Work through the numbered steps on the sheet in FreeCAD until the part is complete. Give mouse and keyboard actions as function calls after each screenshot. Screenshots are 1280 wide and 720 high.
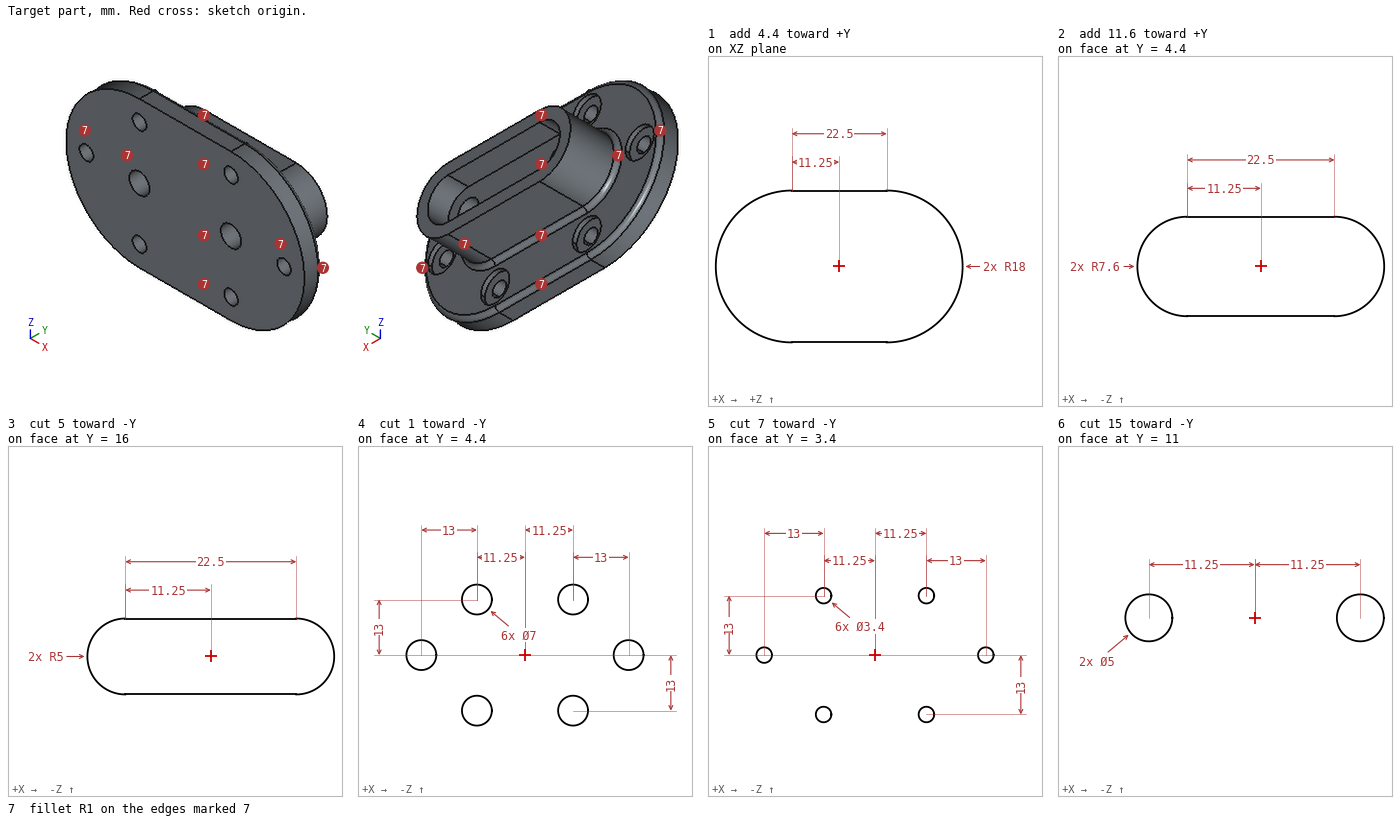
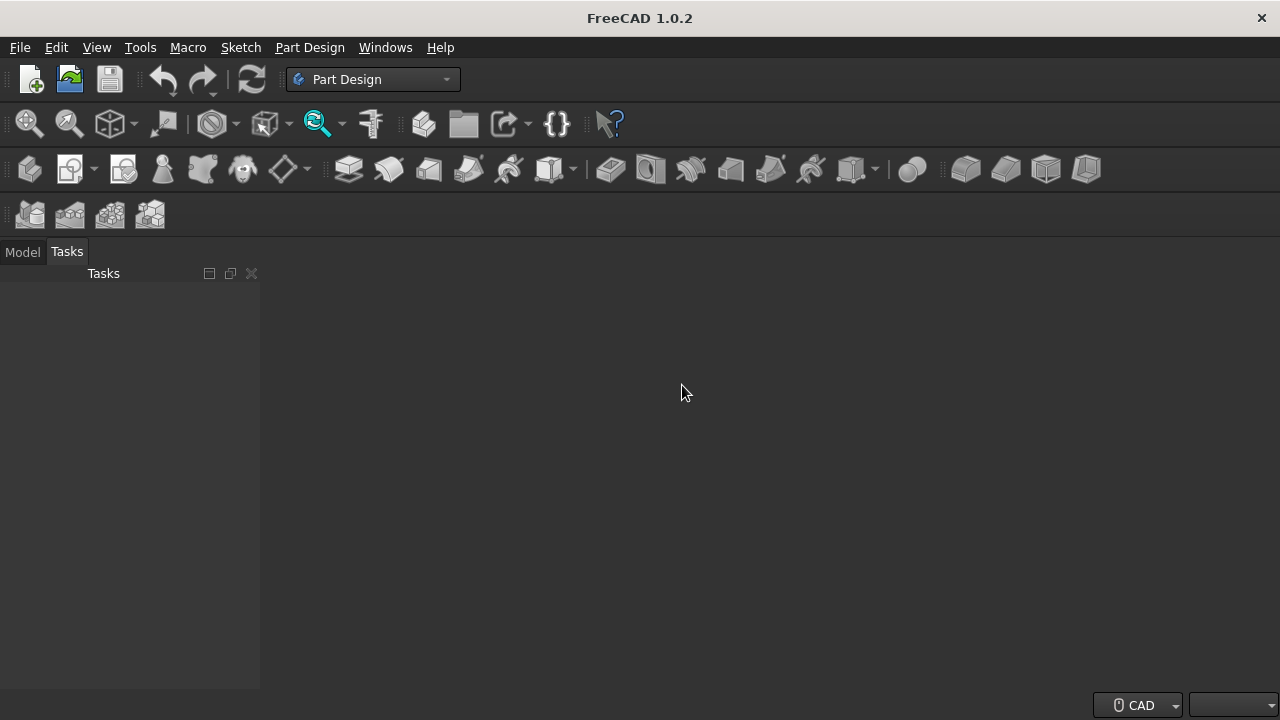
click(30, 80)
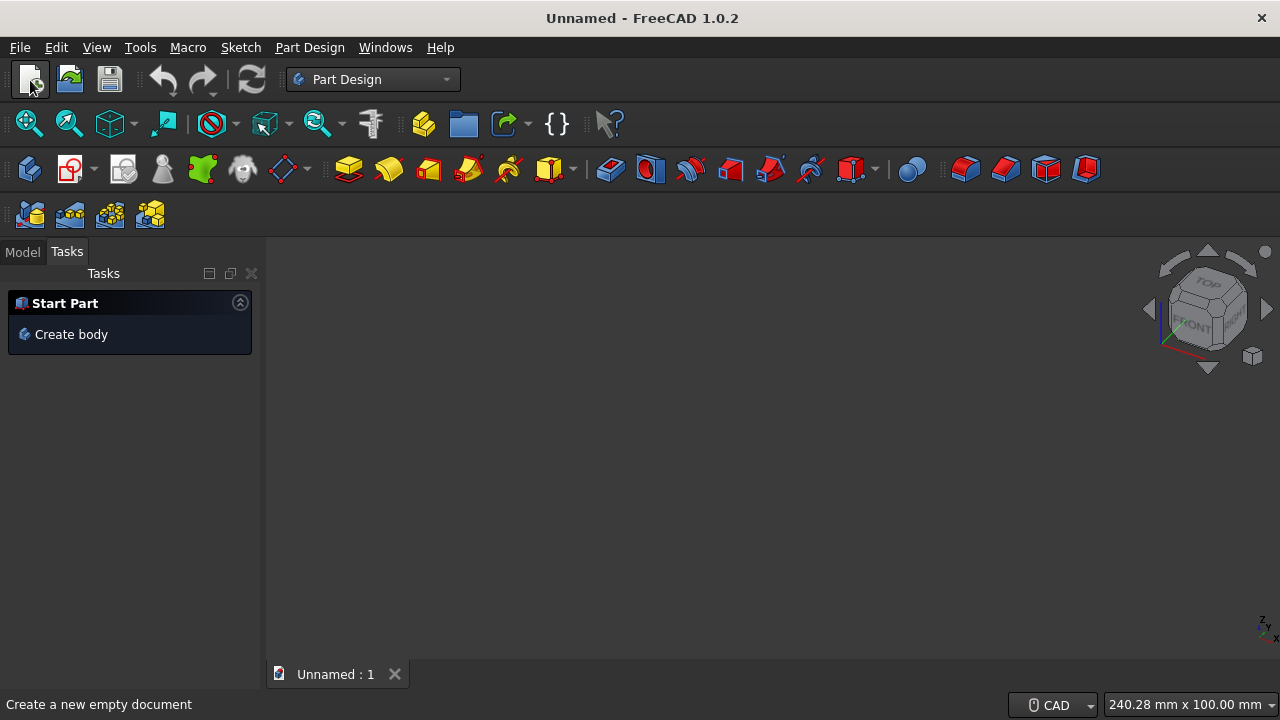
click(70, 170)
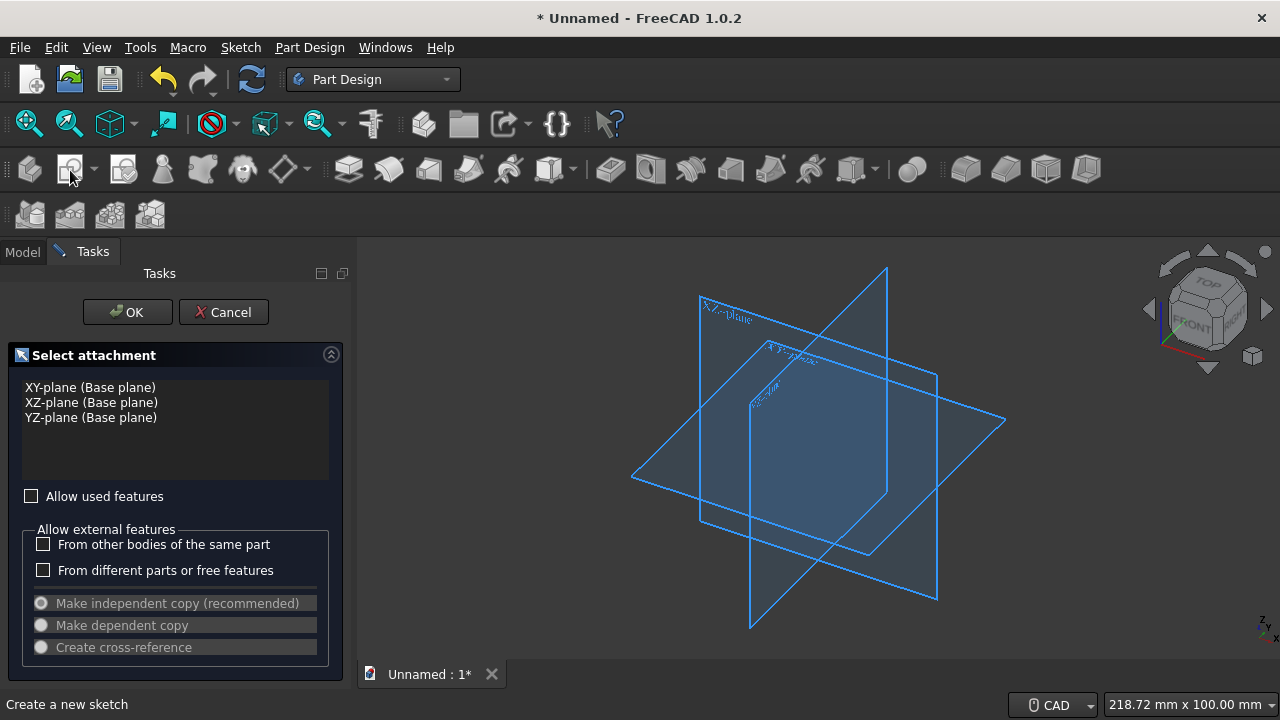
click(82, 402)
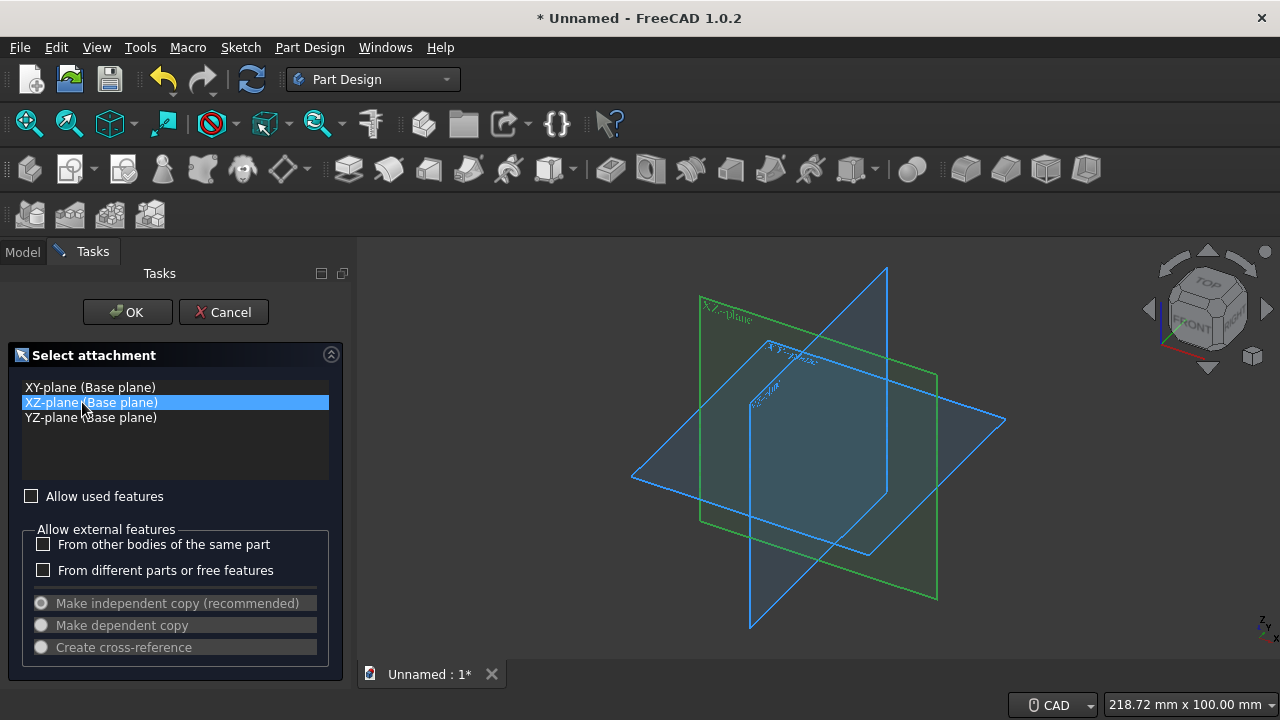
click(128, 312)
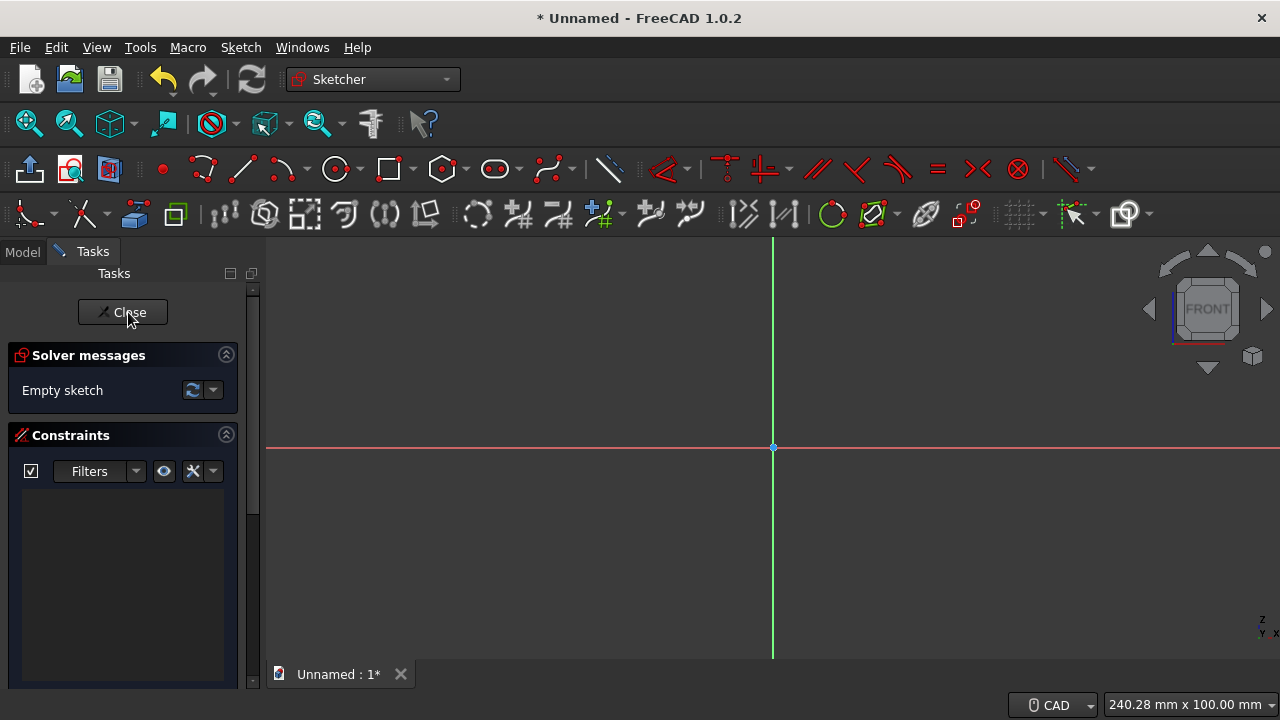
scroll(856, 448, up, 3)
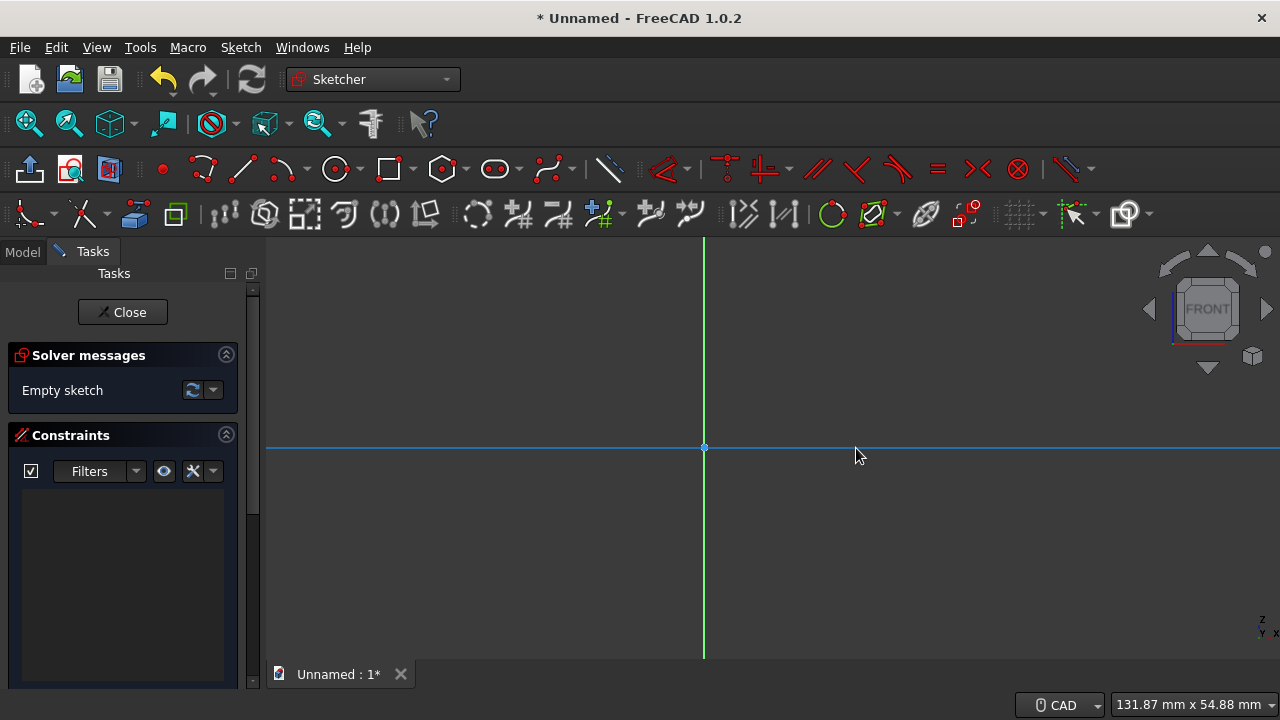
click(496, 170)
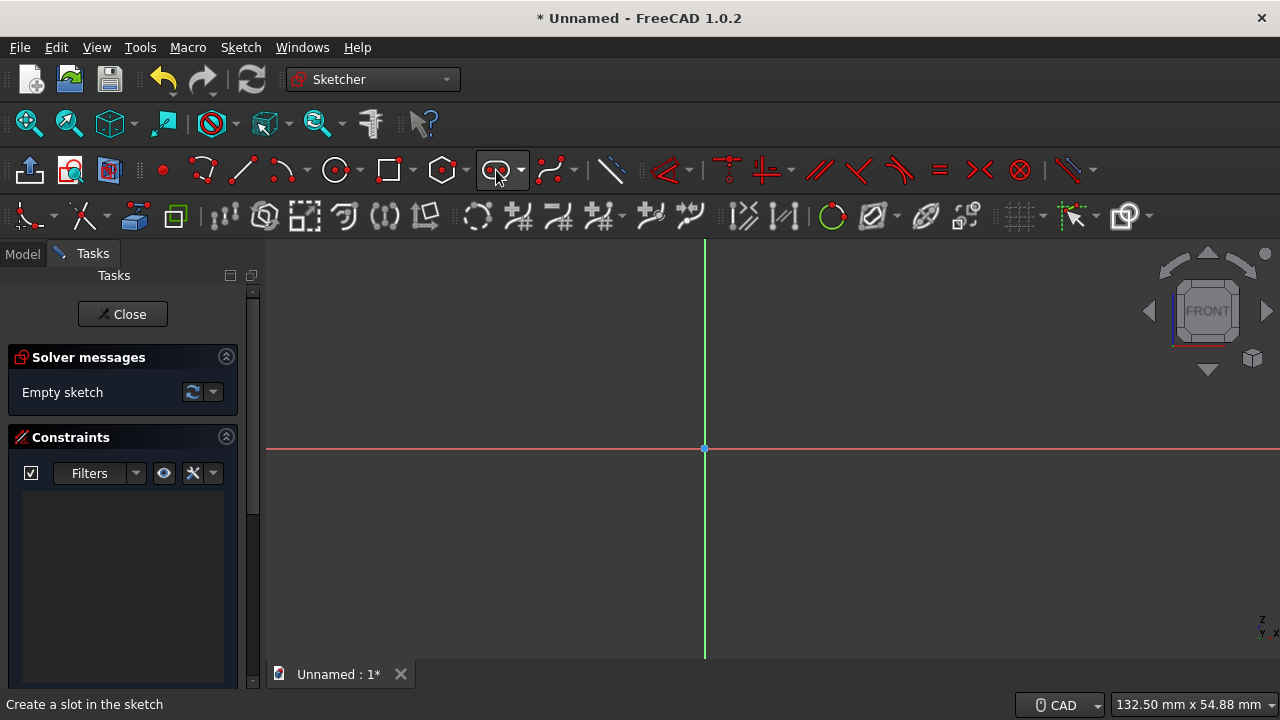
click(619, 449)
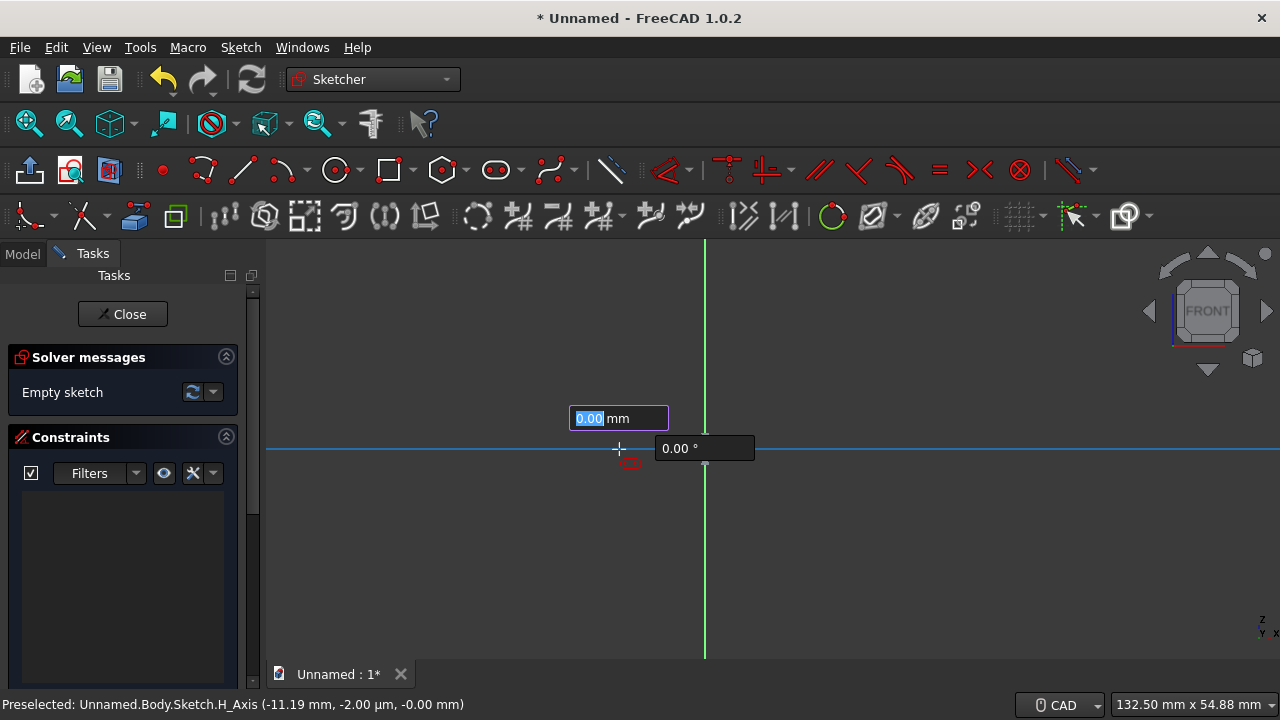
click(791, 440)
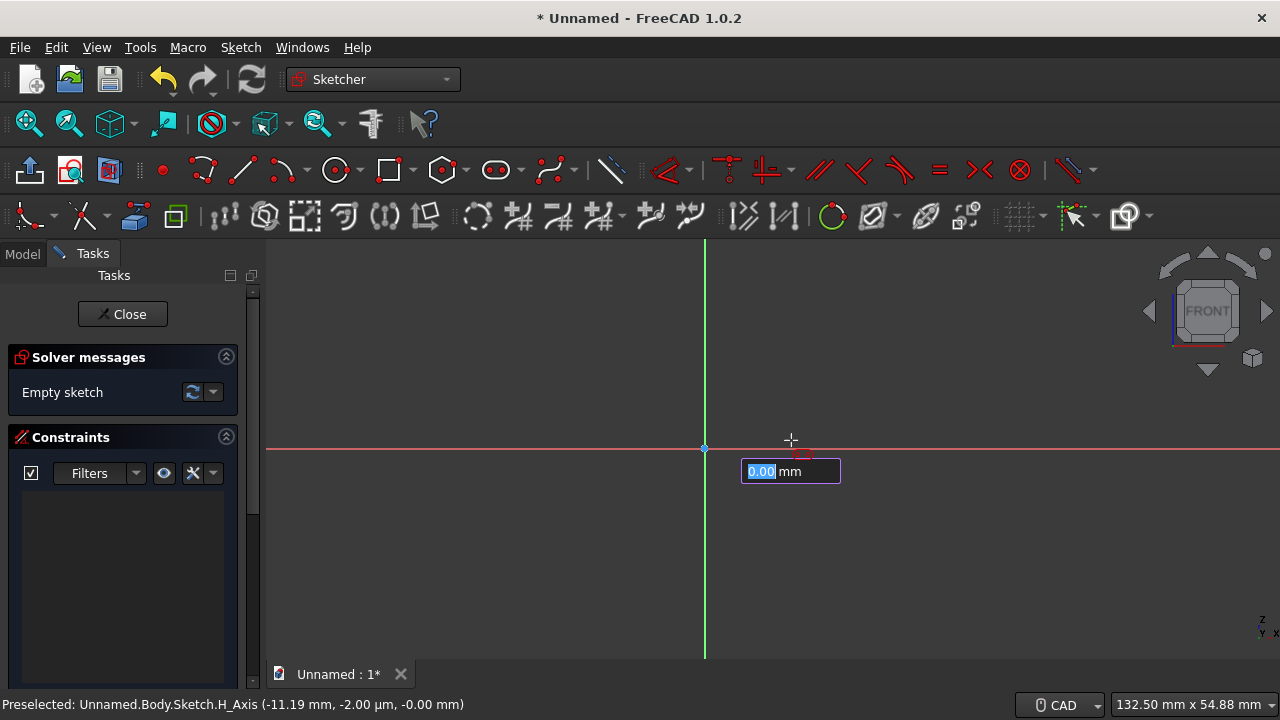
click(679, 311)
key(Escape)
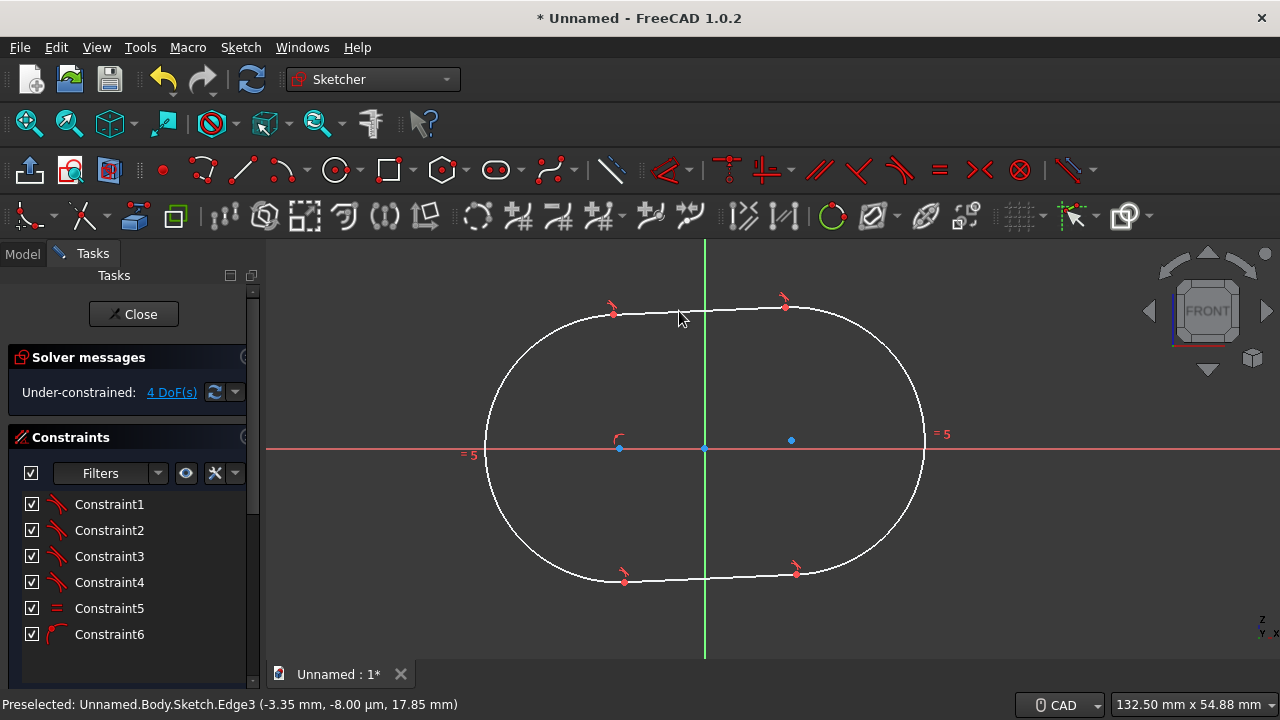
click(665, 313)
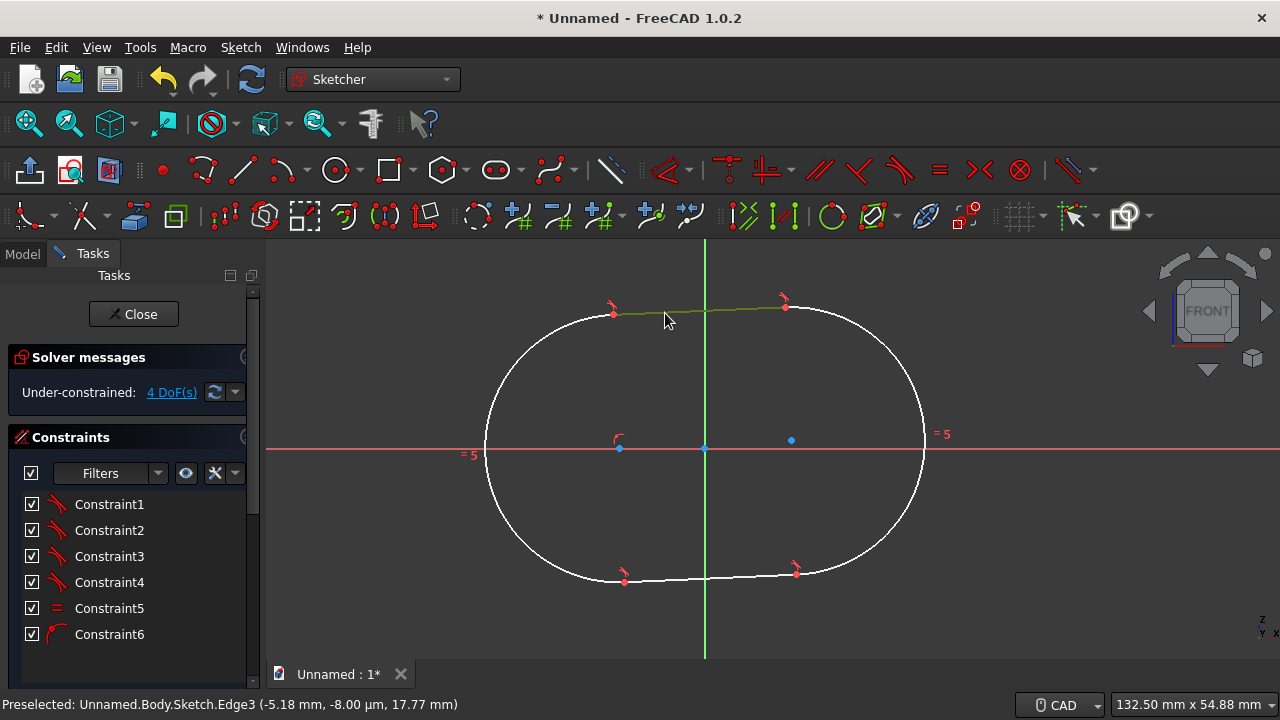
click(794, 170)